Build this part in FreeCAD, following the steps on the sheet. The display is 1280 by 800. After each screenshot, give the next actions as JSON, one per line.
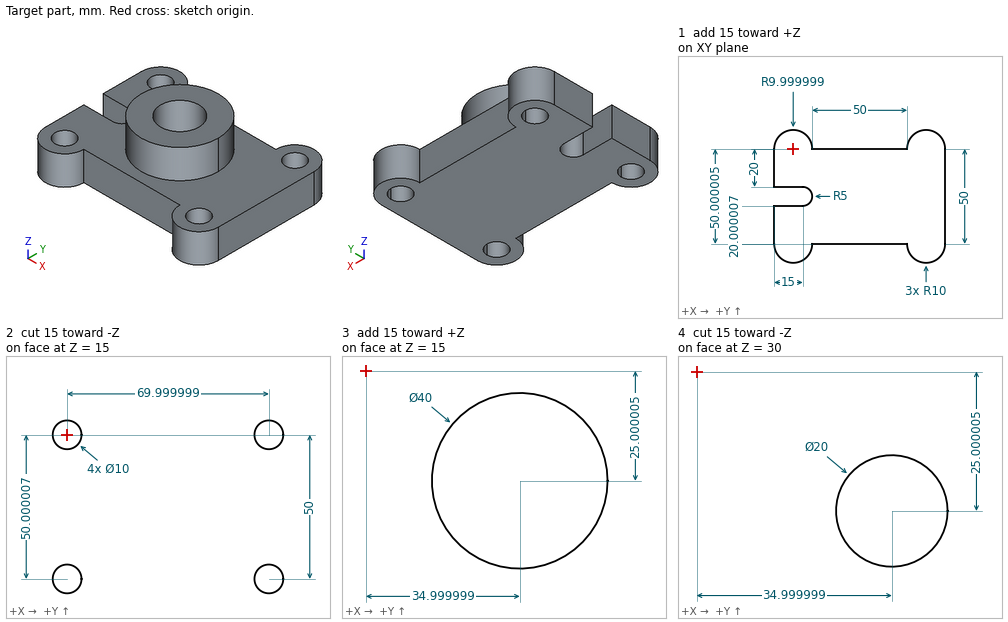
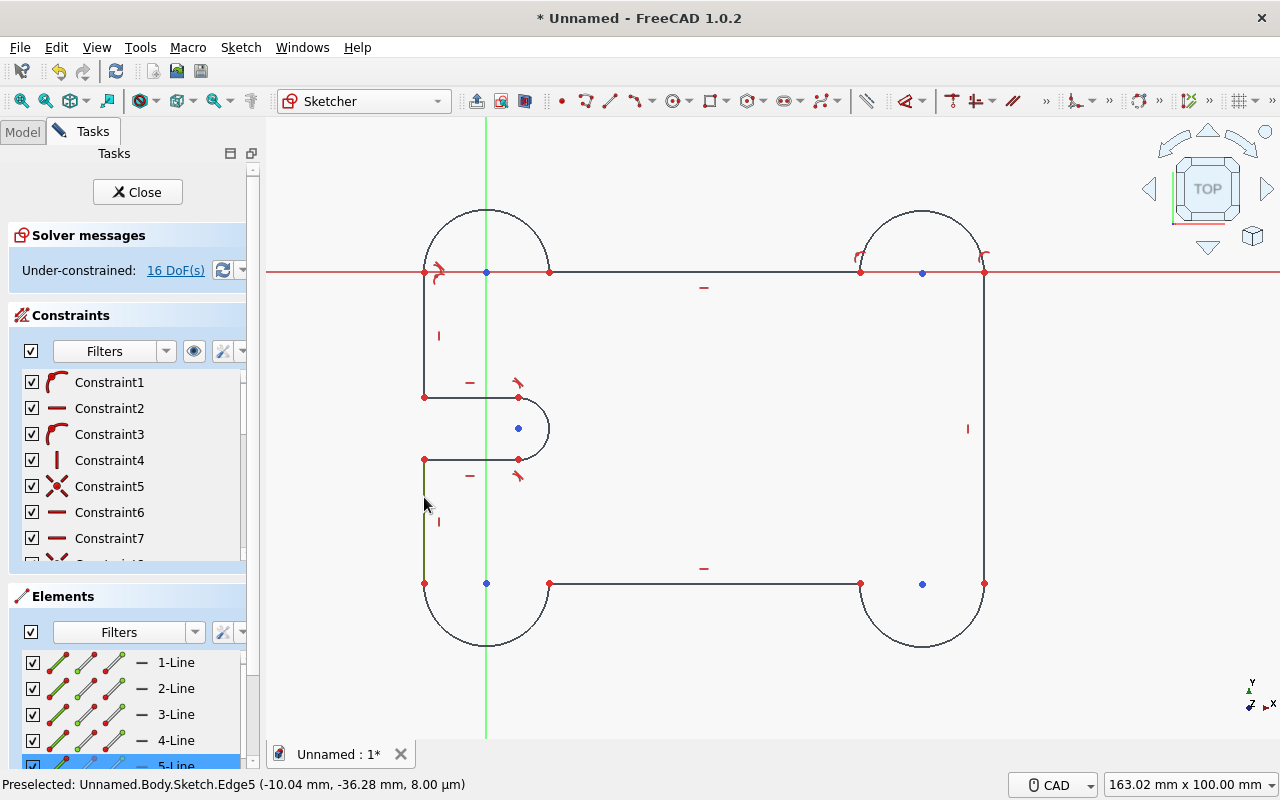
{"action": "left_click", "coordinate": [450, 634]}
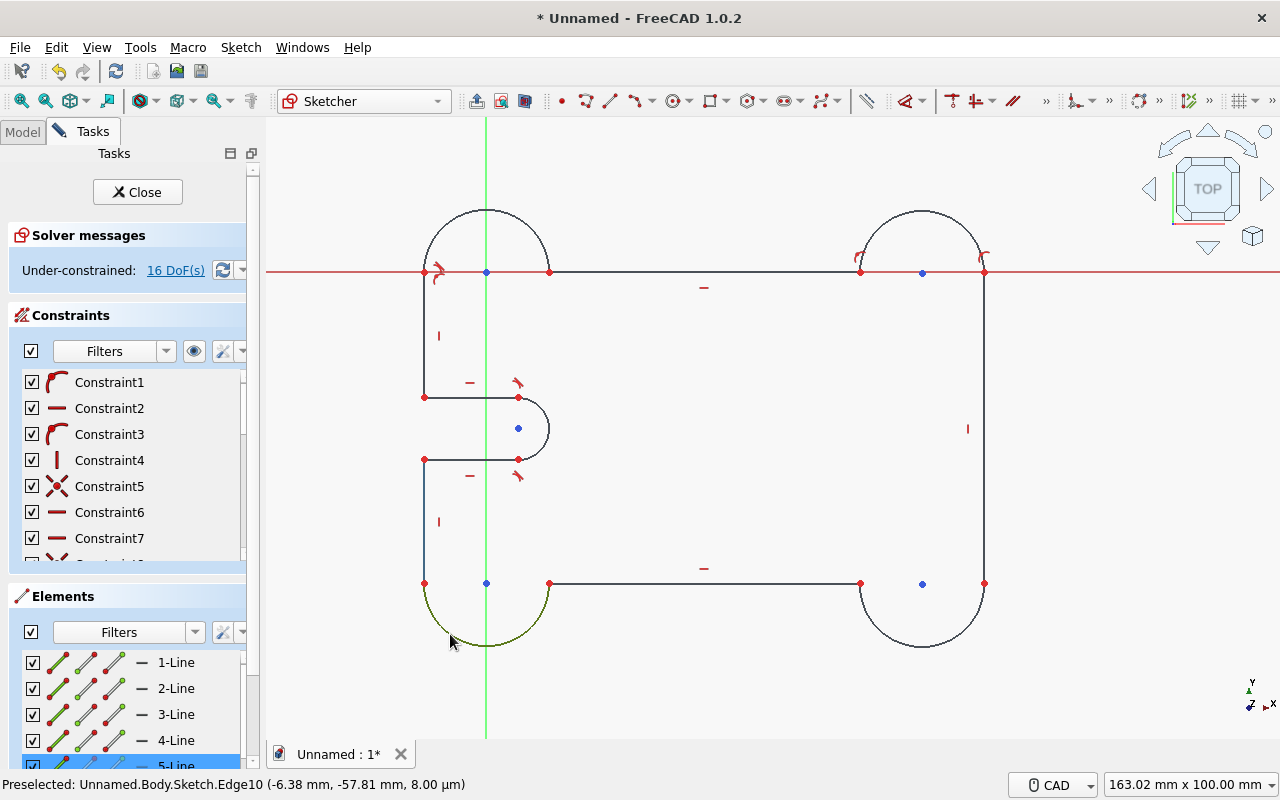
{"action": "key", "text": "t"}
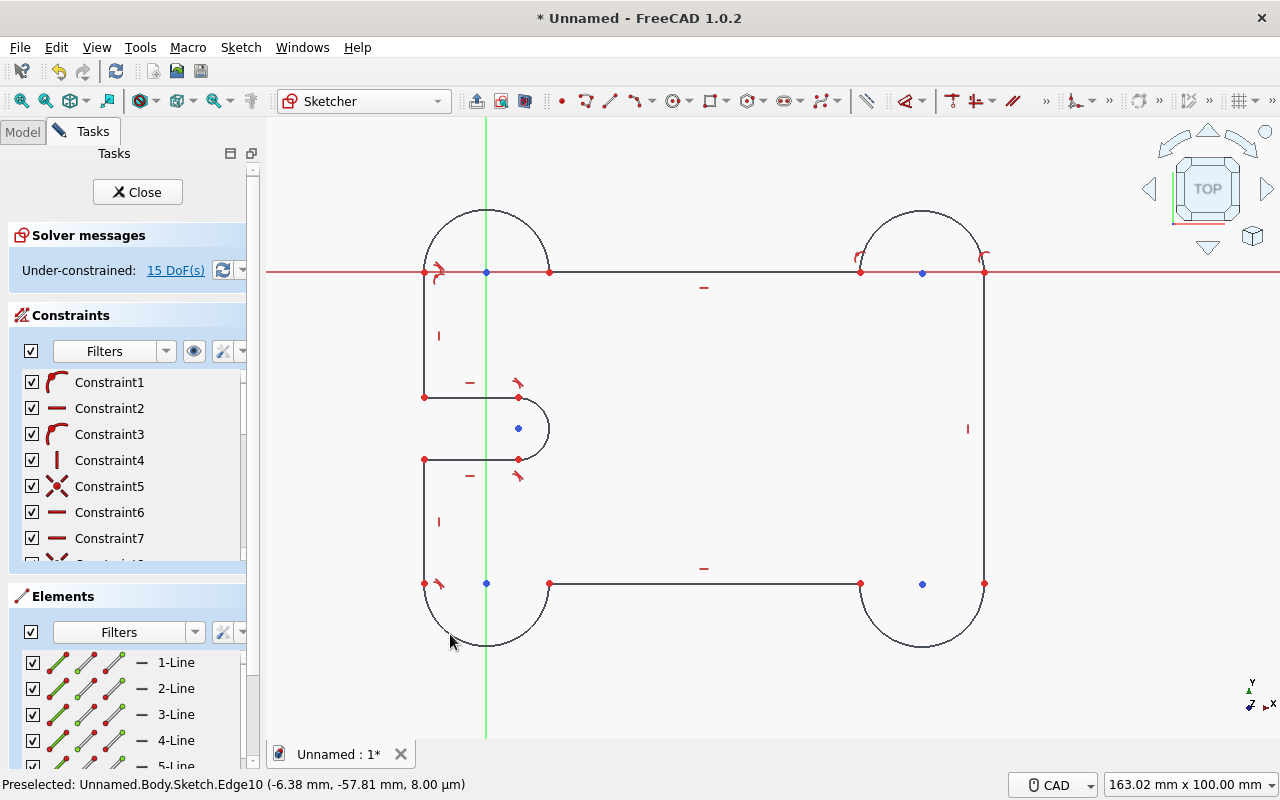
{"action": "left_click", "coordinate": [984, 490]}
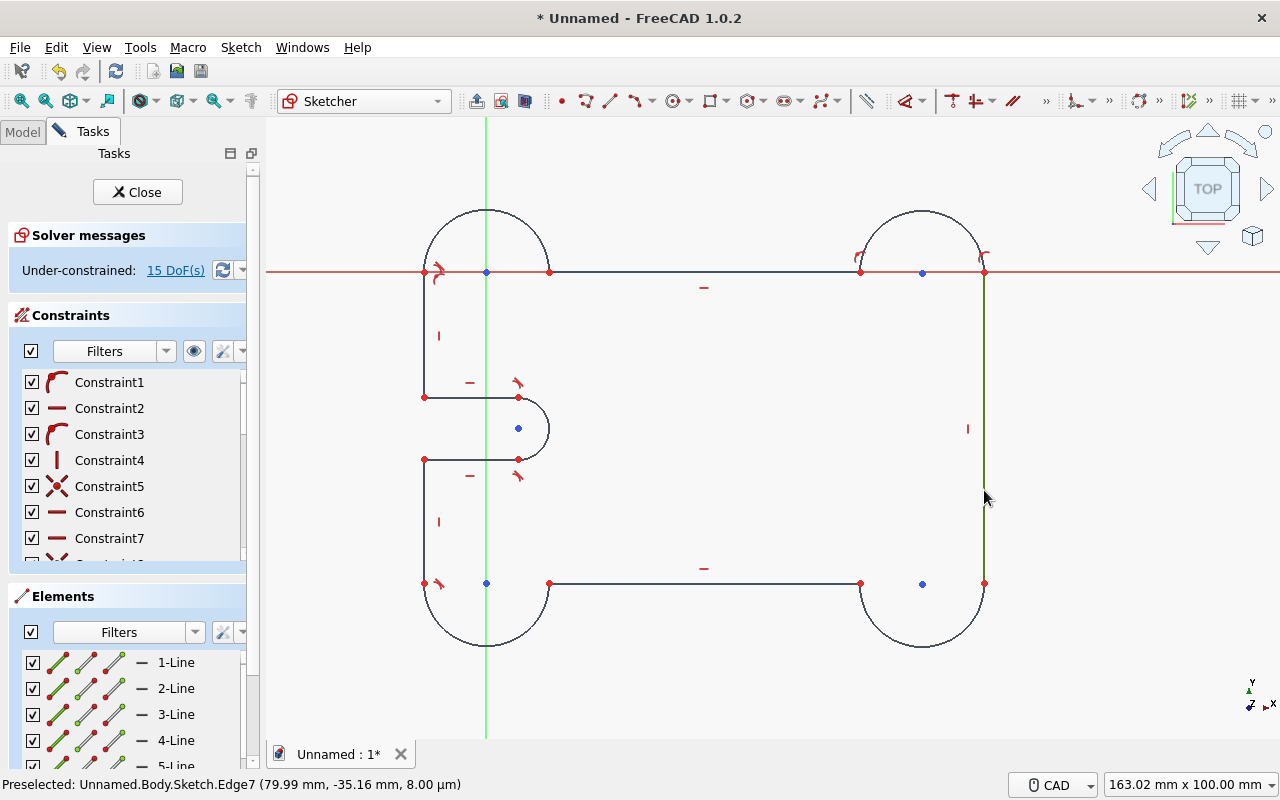
{"action": "left_click", "coordinate": [885, 635]}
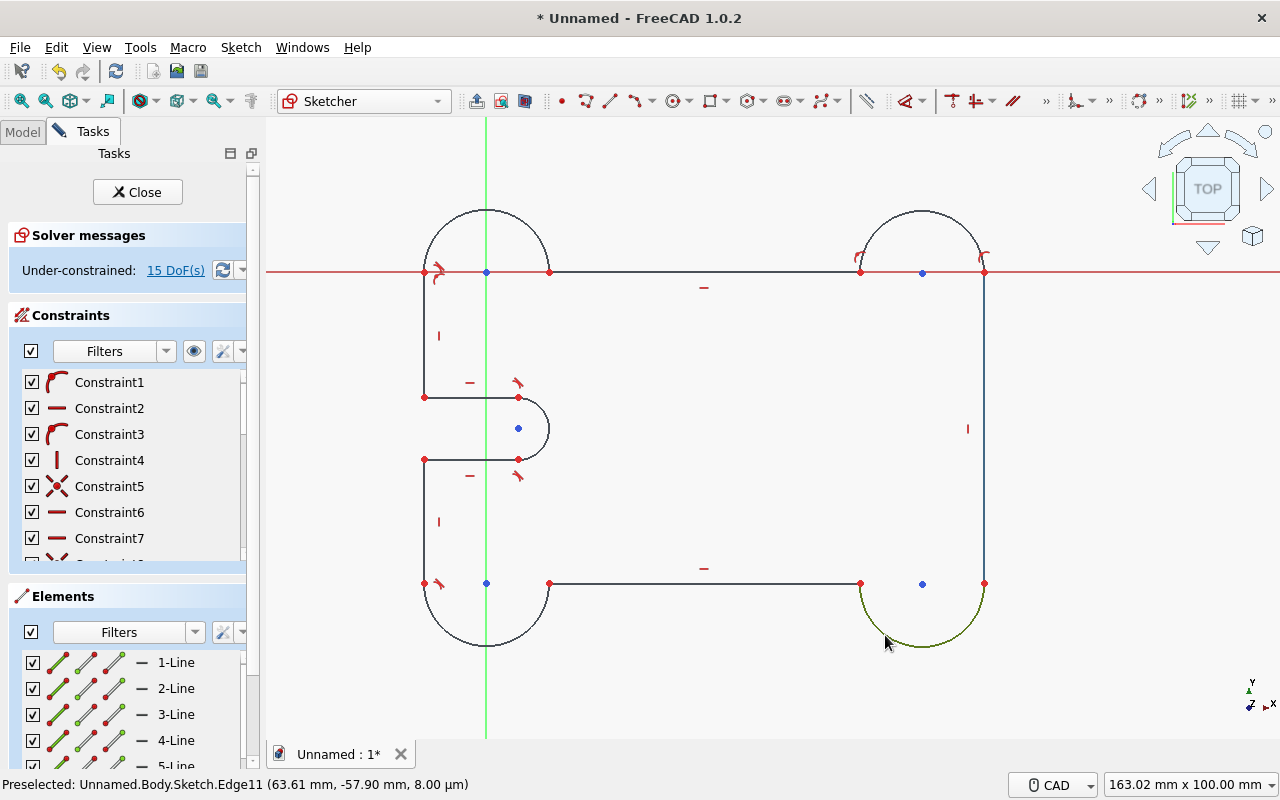
{"action": "key", "text": "t"}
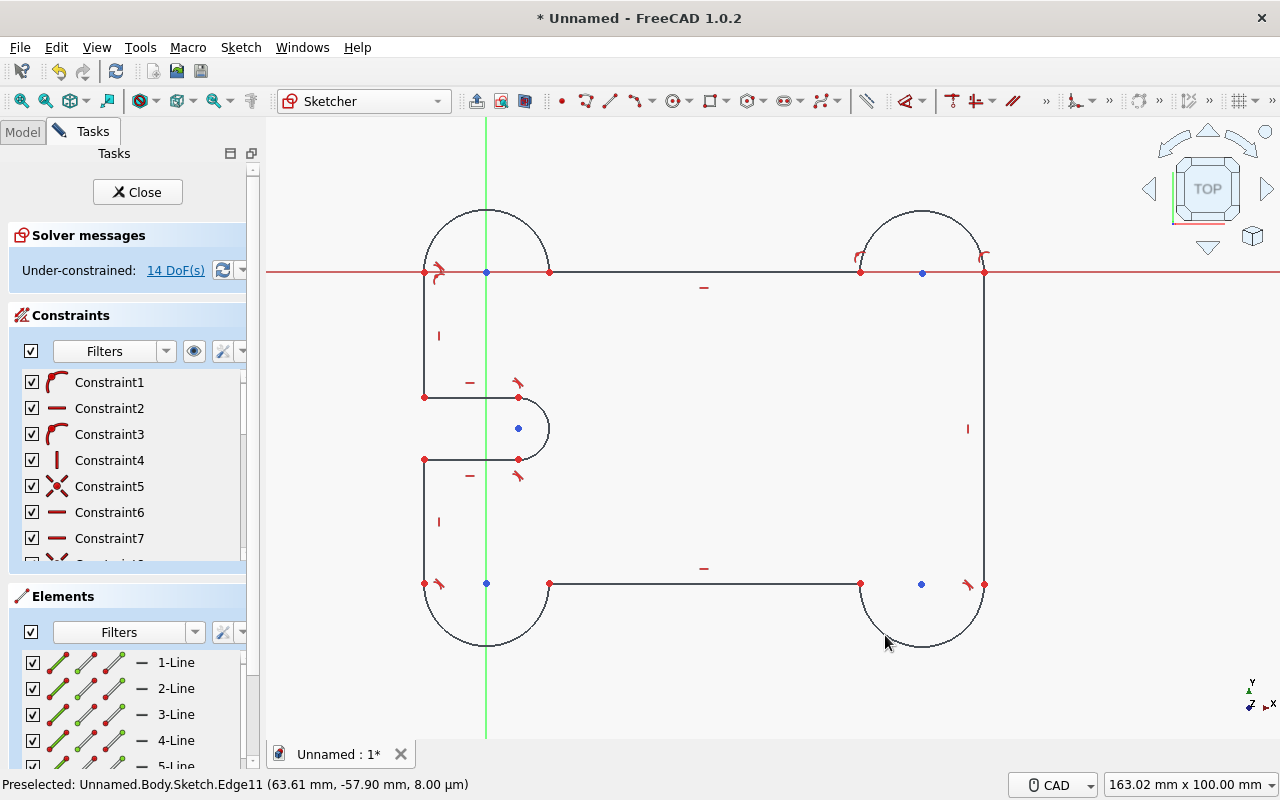
{"action": "left_click", "coordinate": [984, 491]}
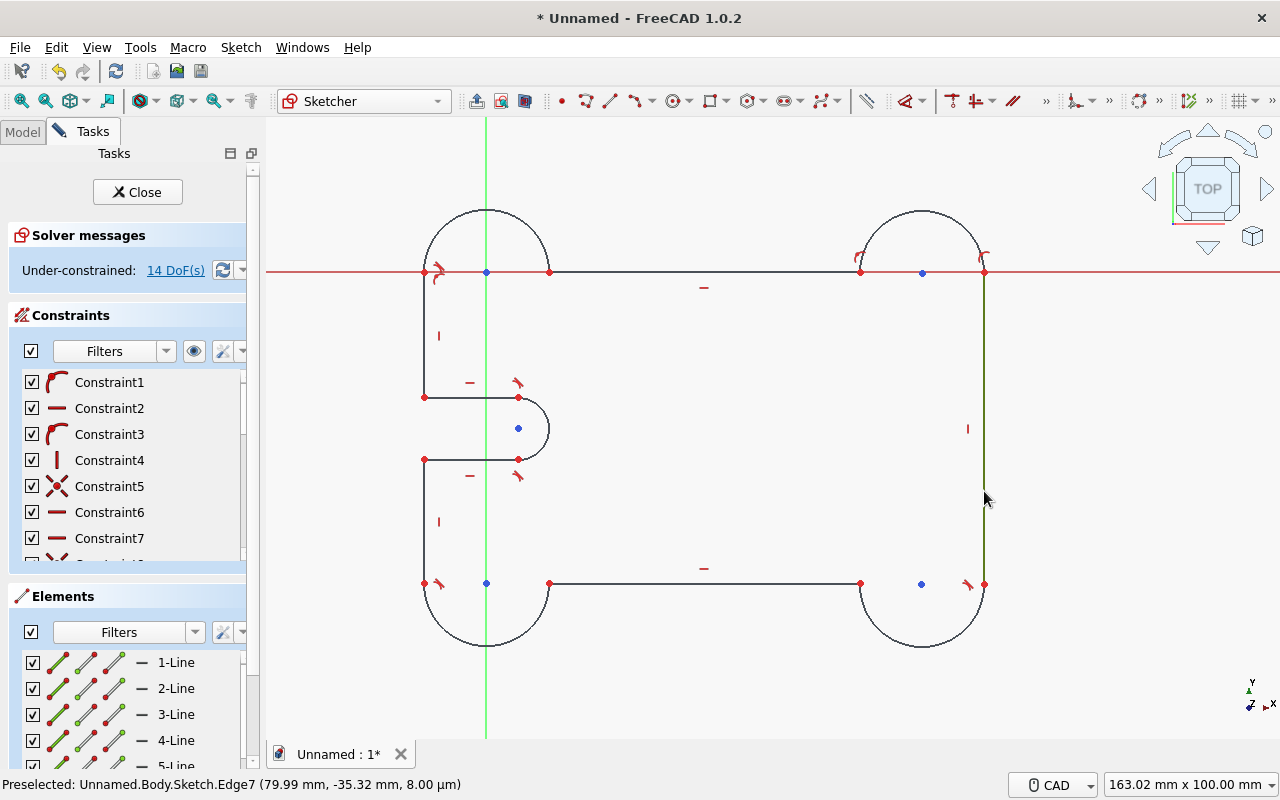
{"action": "left_click", "coordinate": [958, 223]}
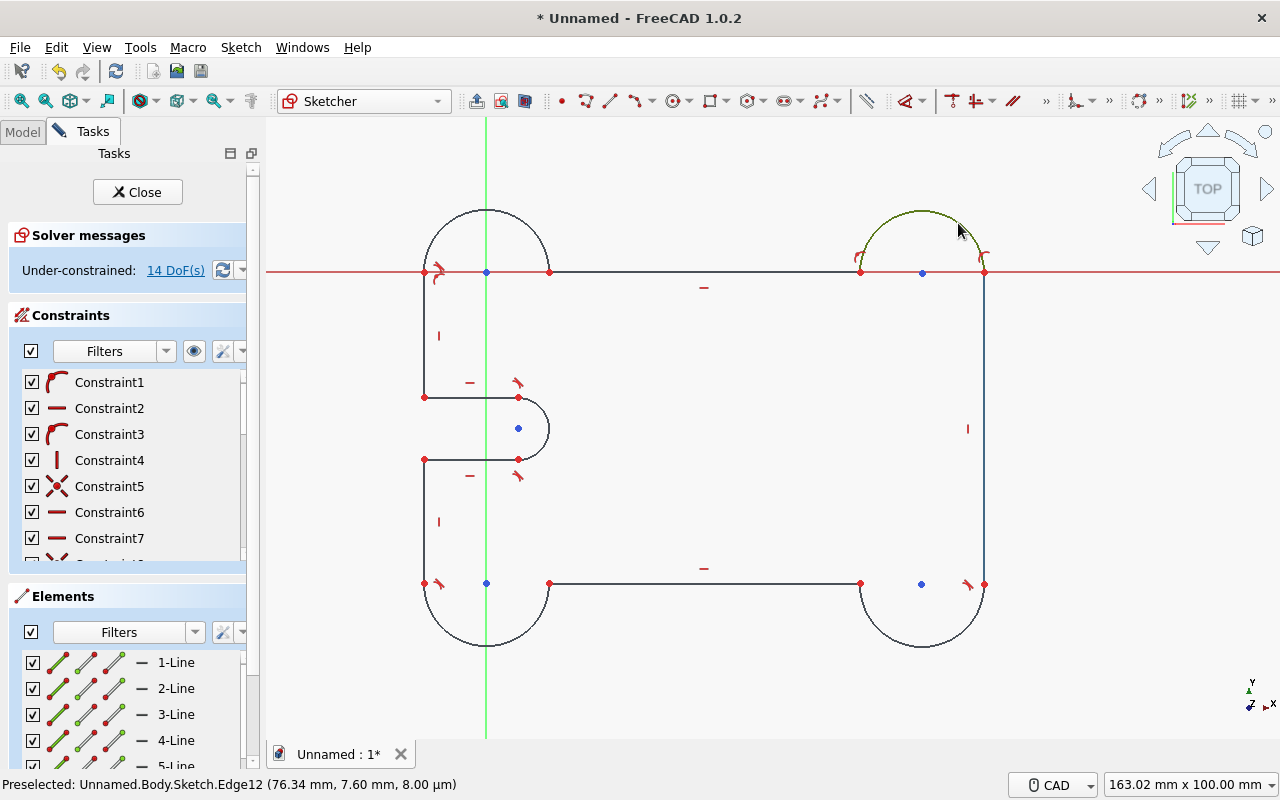
{"action": "key", "text": "t"}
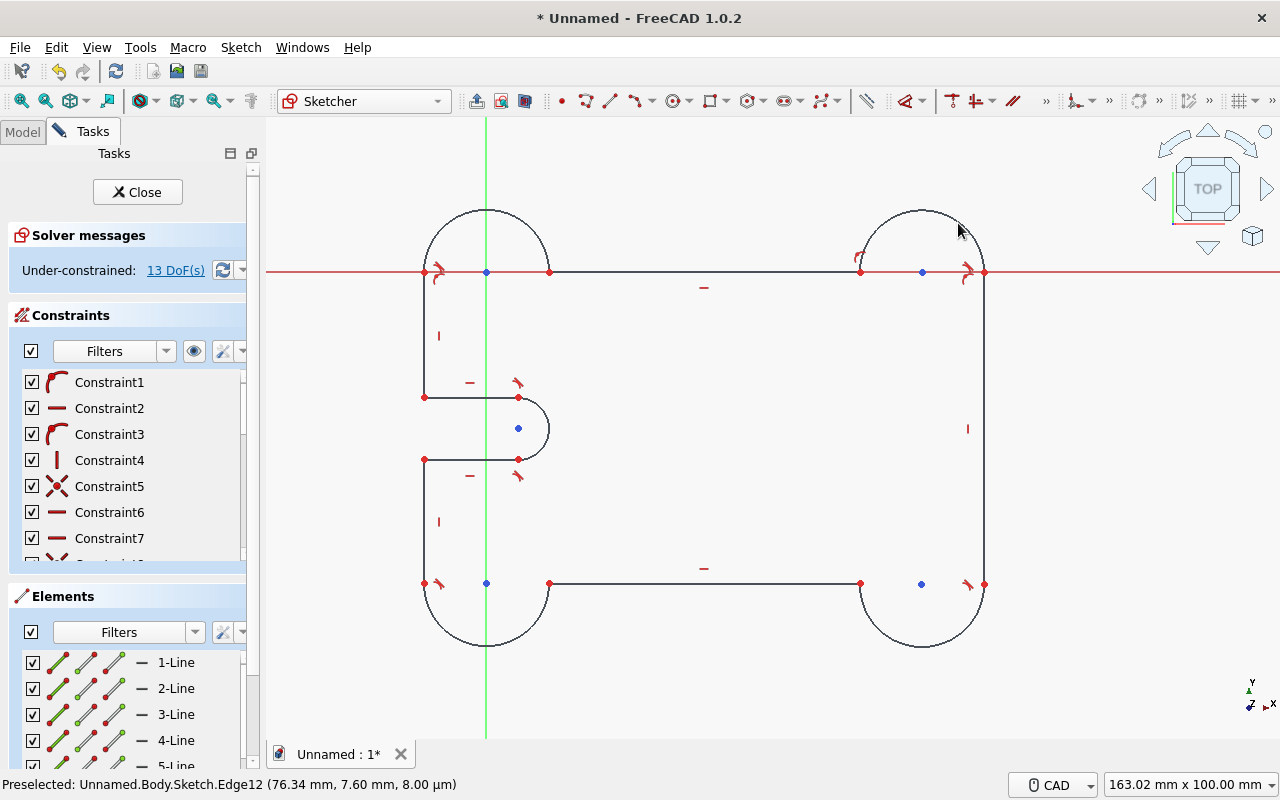
{"action": "left_click", "coordinate": [450, 634]}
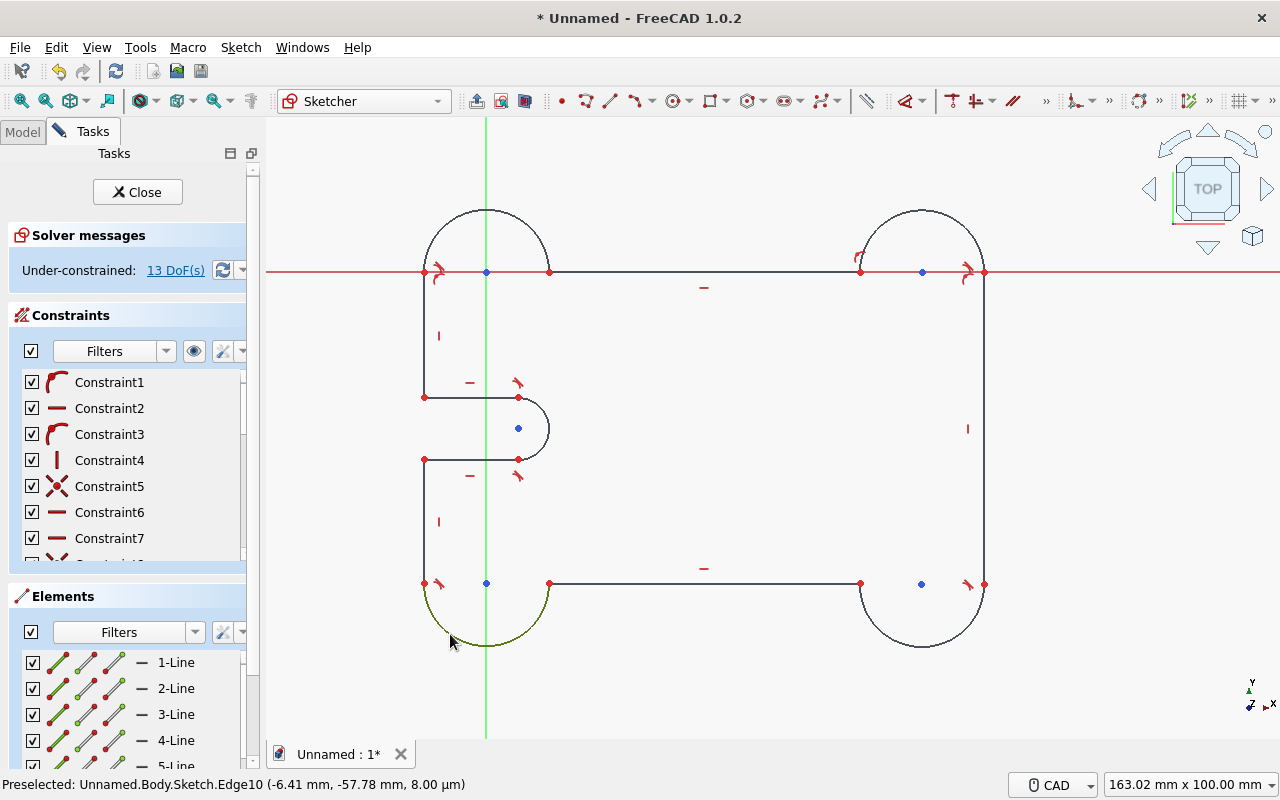
{"action": "left_click", "coordinate": [885, 635]}